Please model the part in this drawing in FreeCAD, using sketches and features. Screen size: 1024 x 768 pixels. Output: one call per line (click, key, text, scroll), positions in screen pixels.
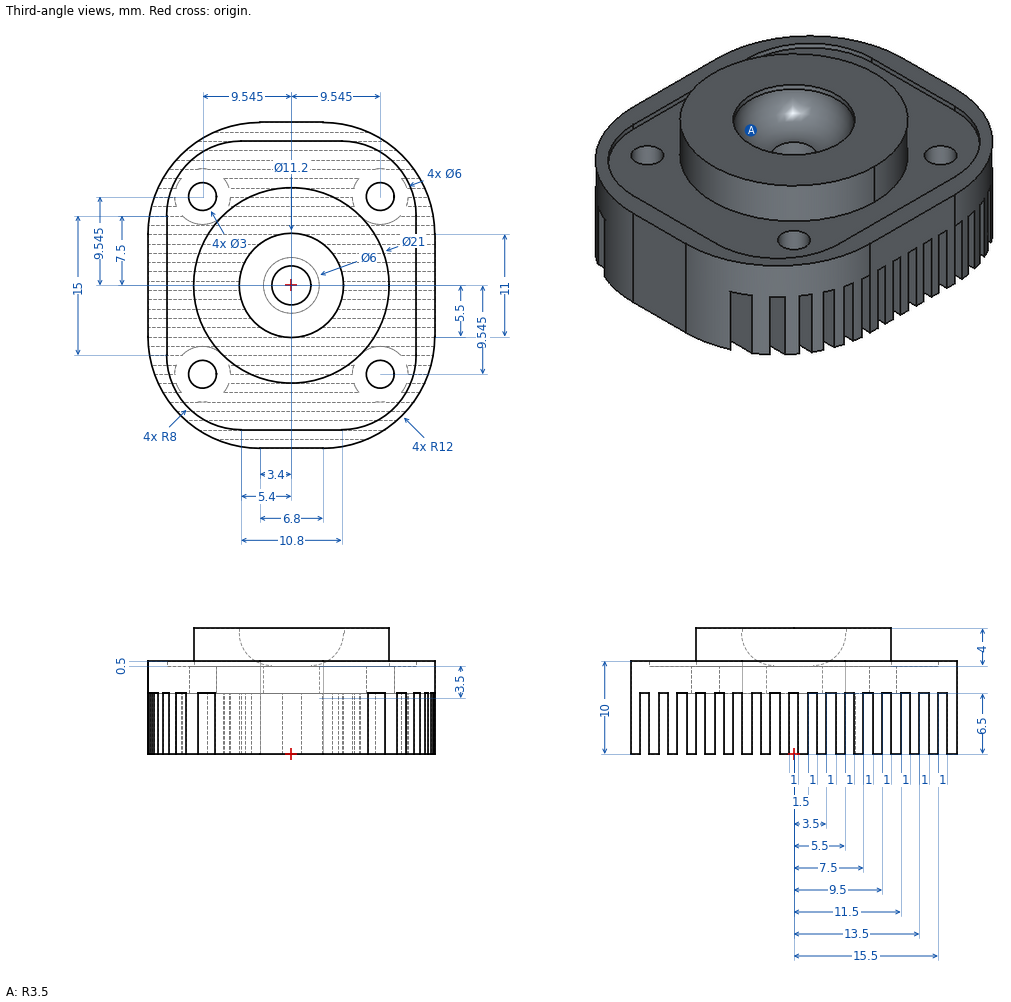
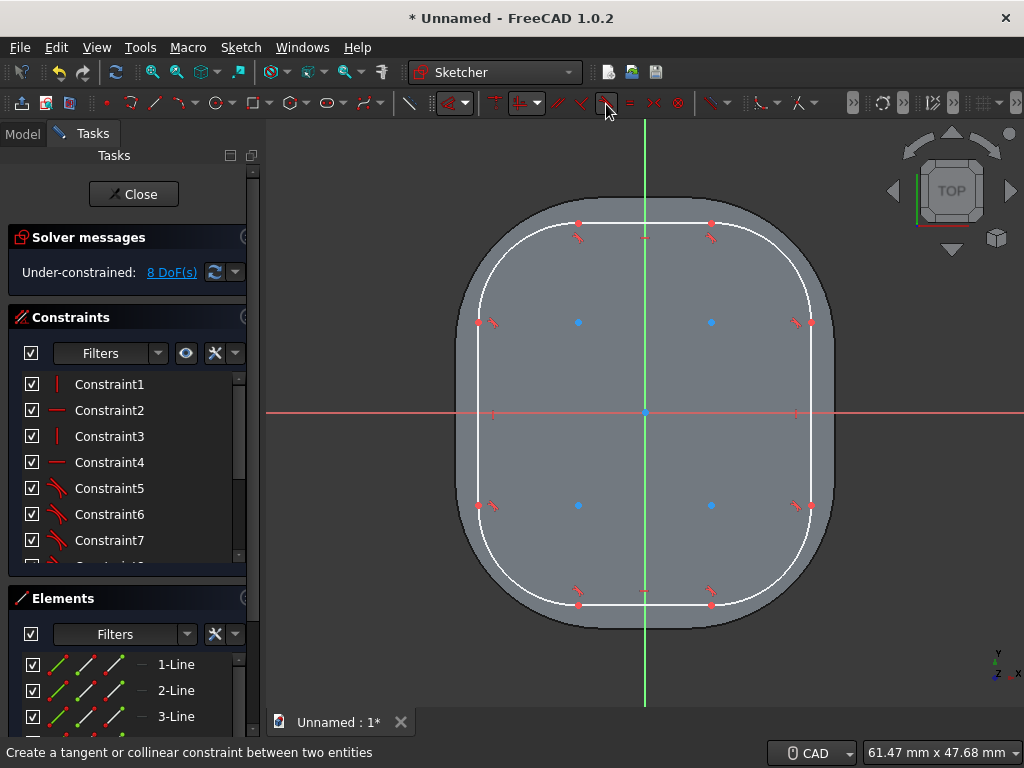
click(489, 551)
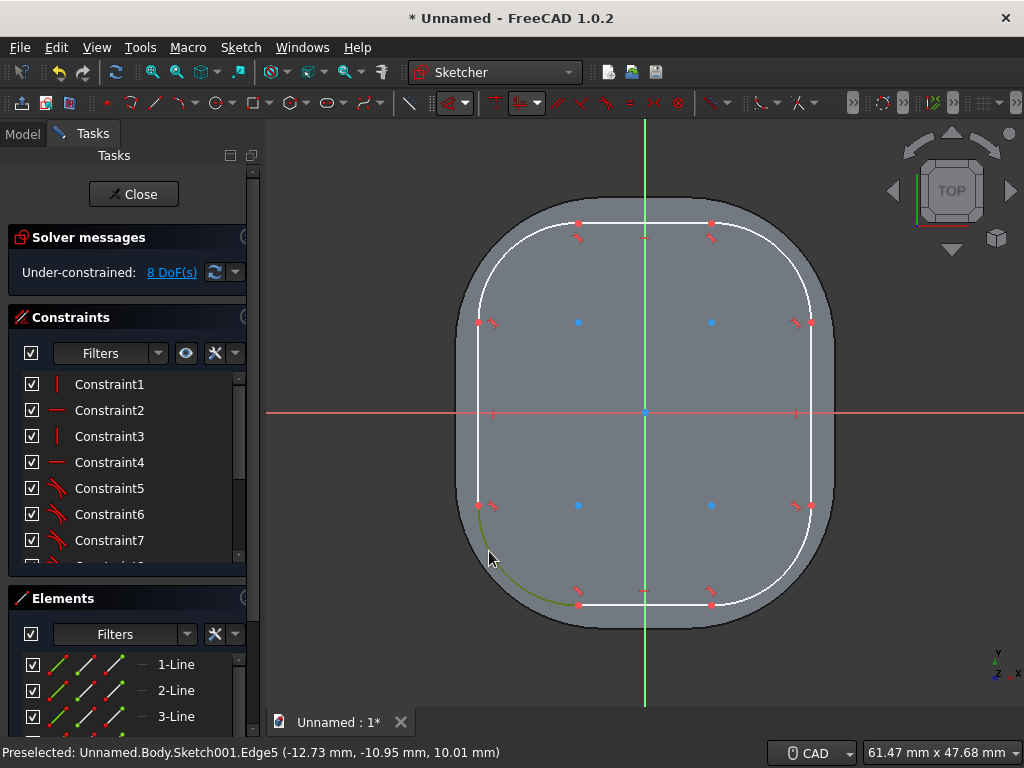
click(757, 595)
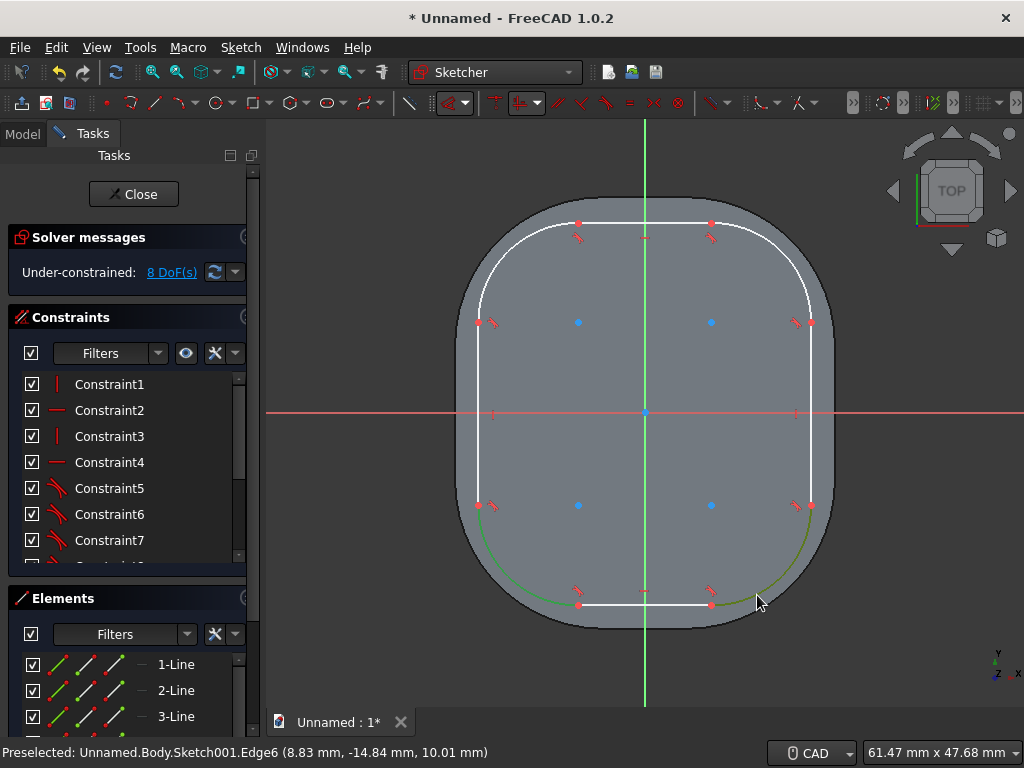
click(800, 277)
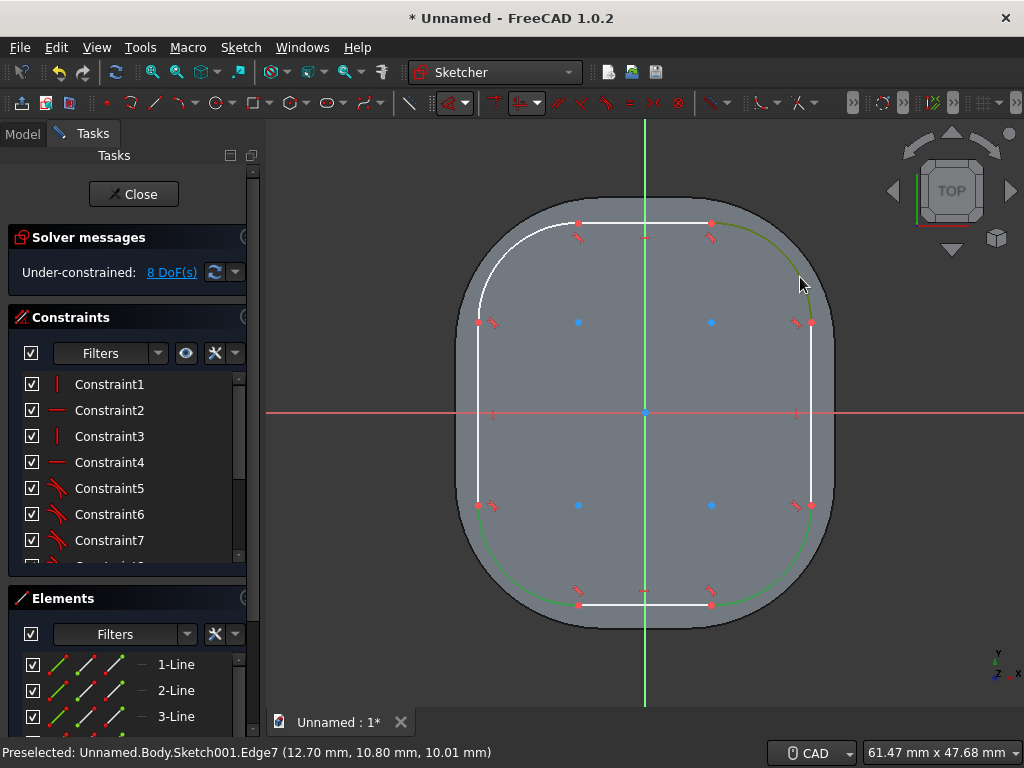
click(533, 234)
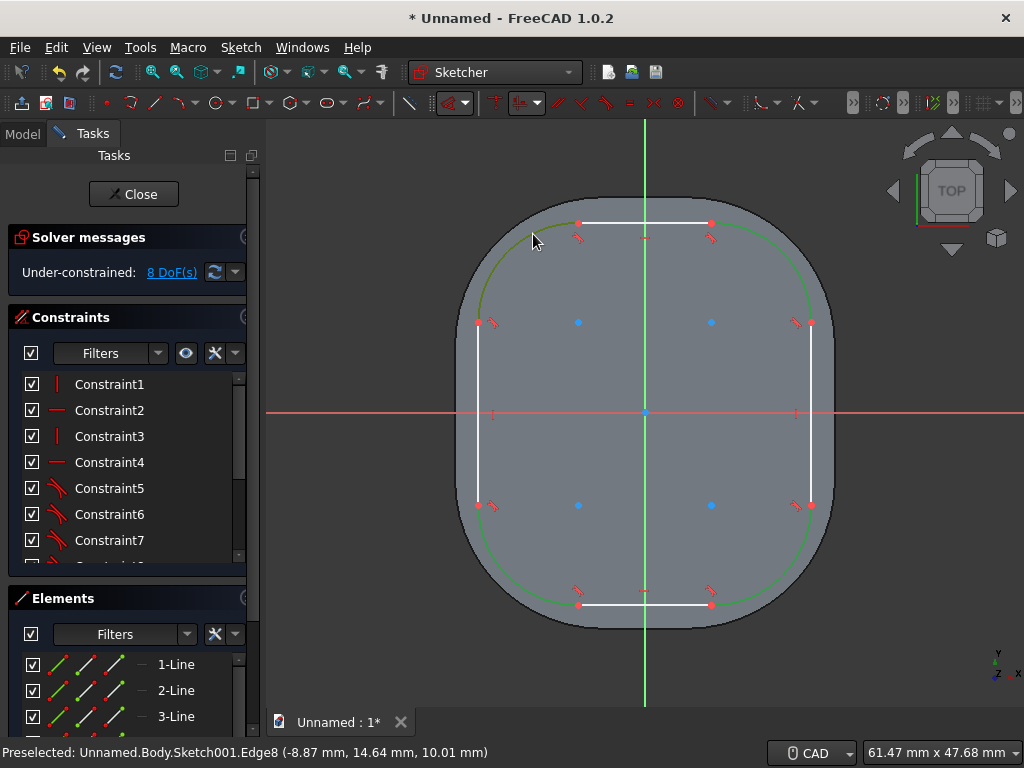
click(630, 104)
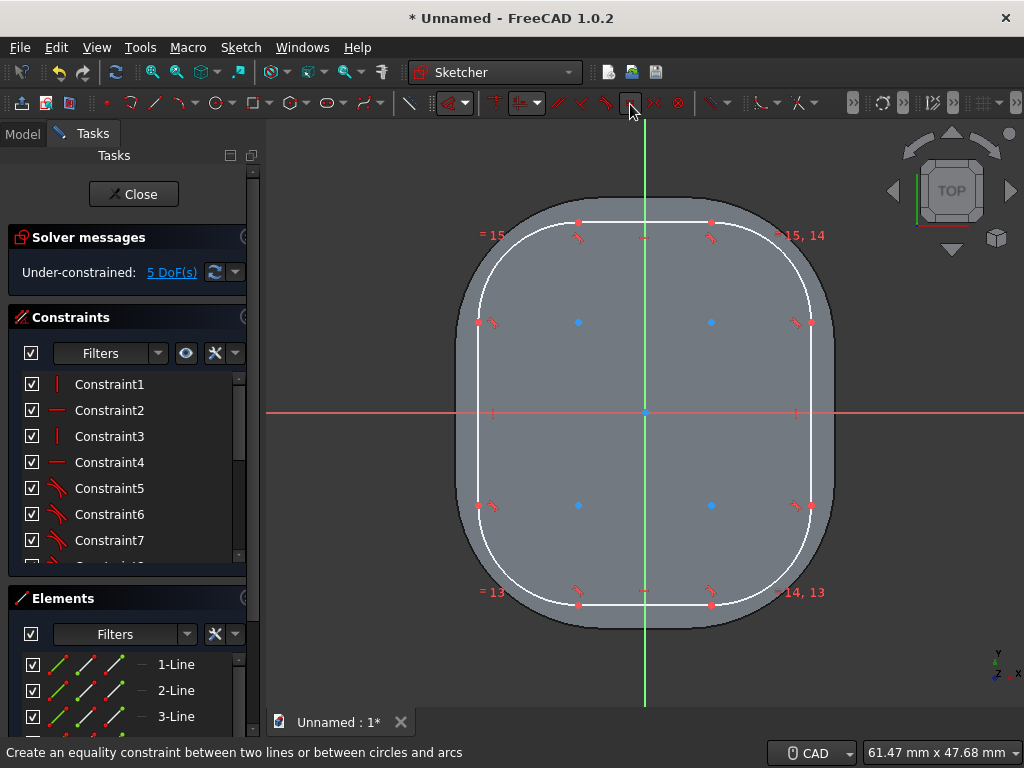
click(489, 551)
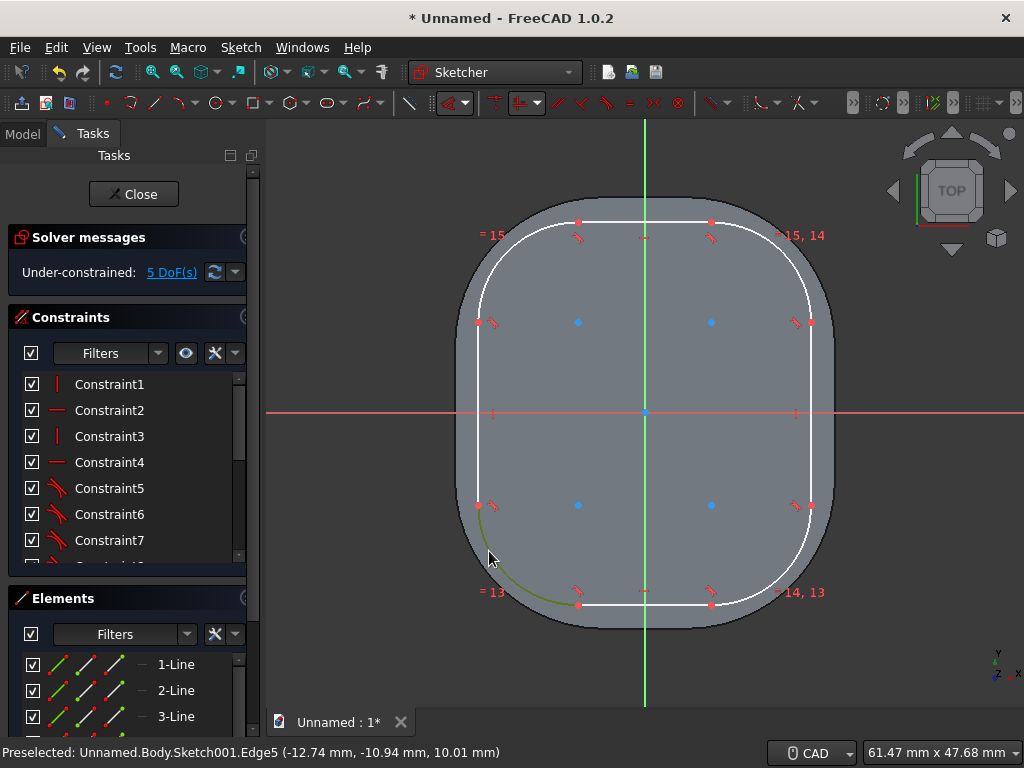
click(468, 104)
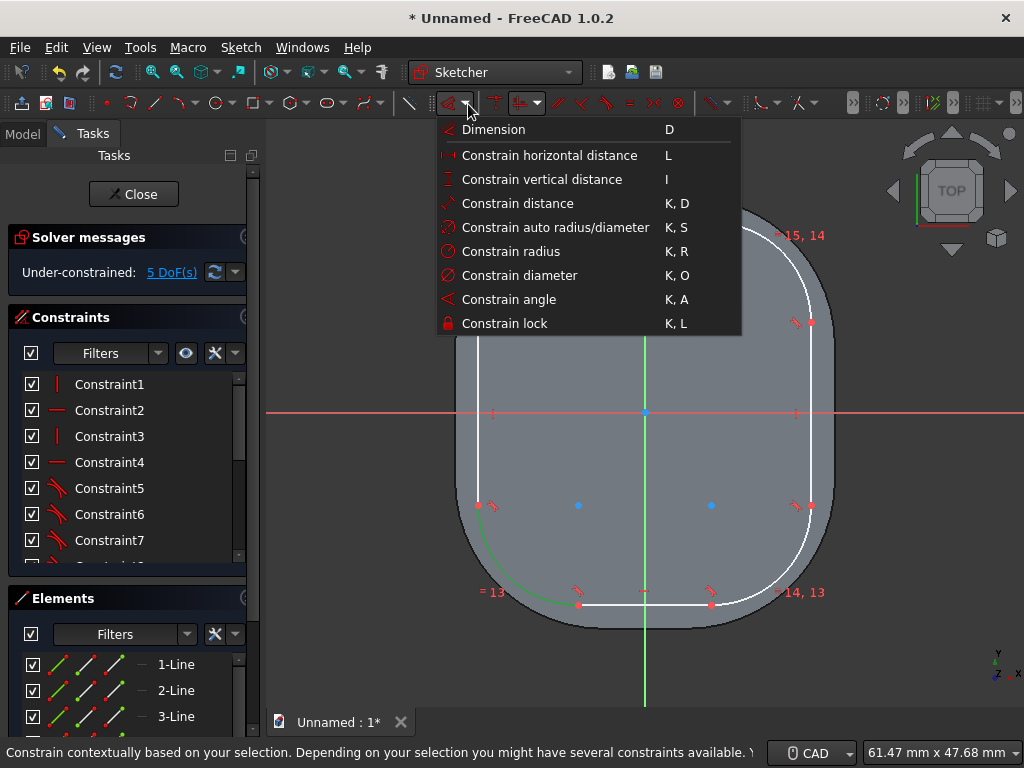
click(589, 251)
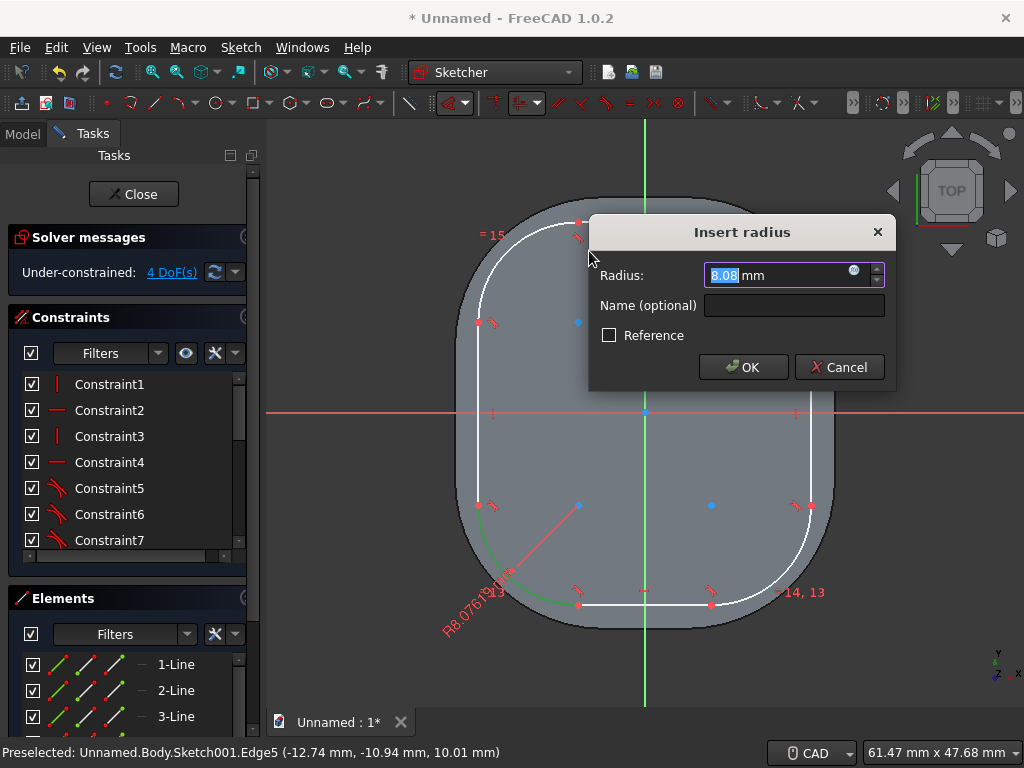
text(8)
key(Return)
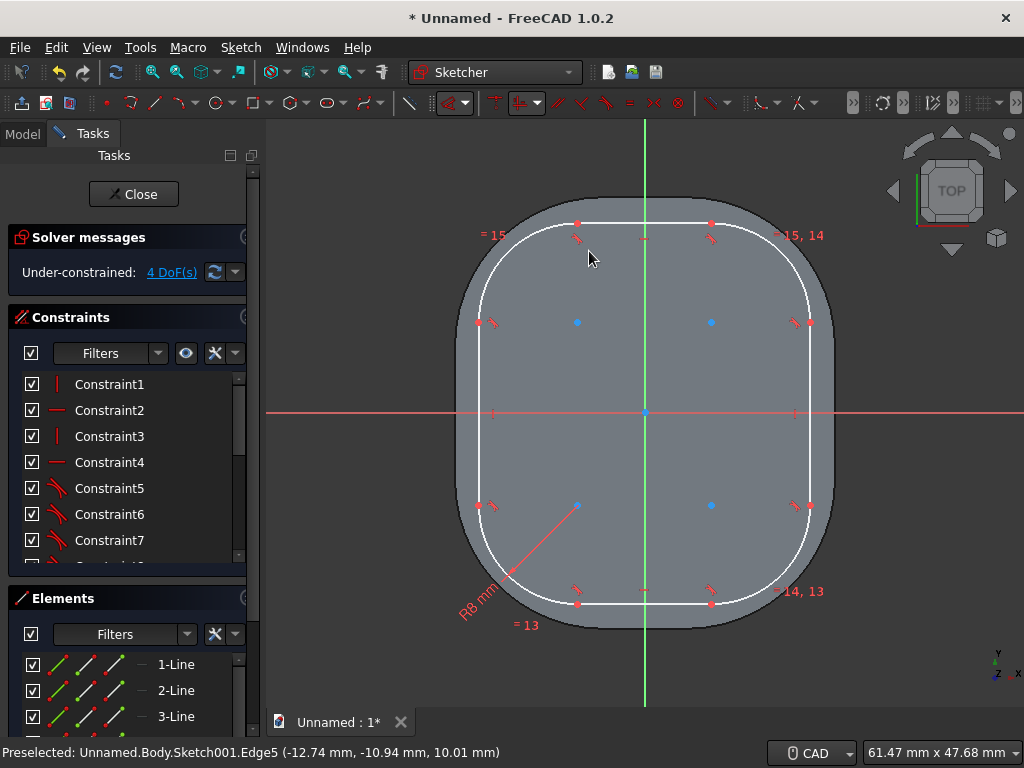
click(479, 377)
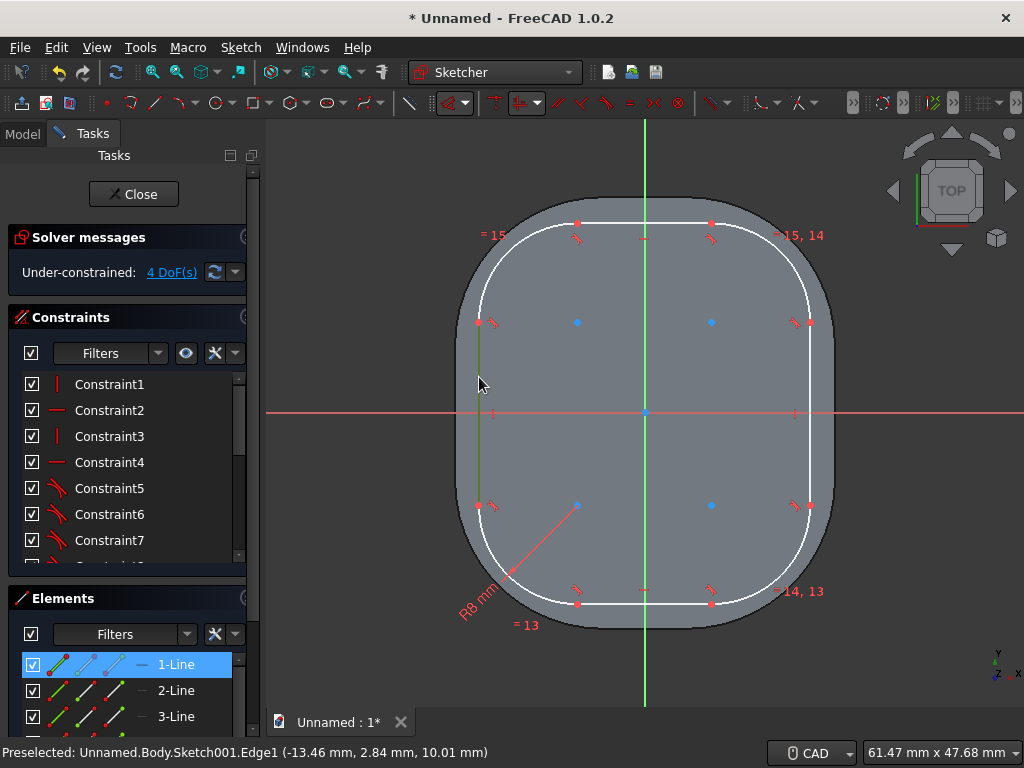
click(468, 104)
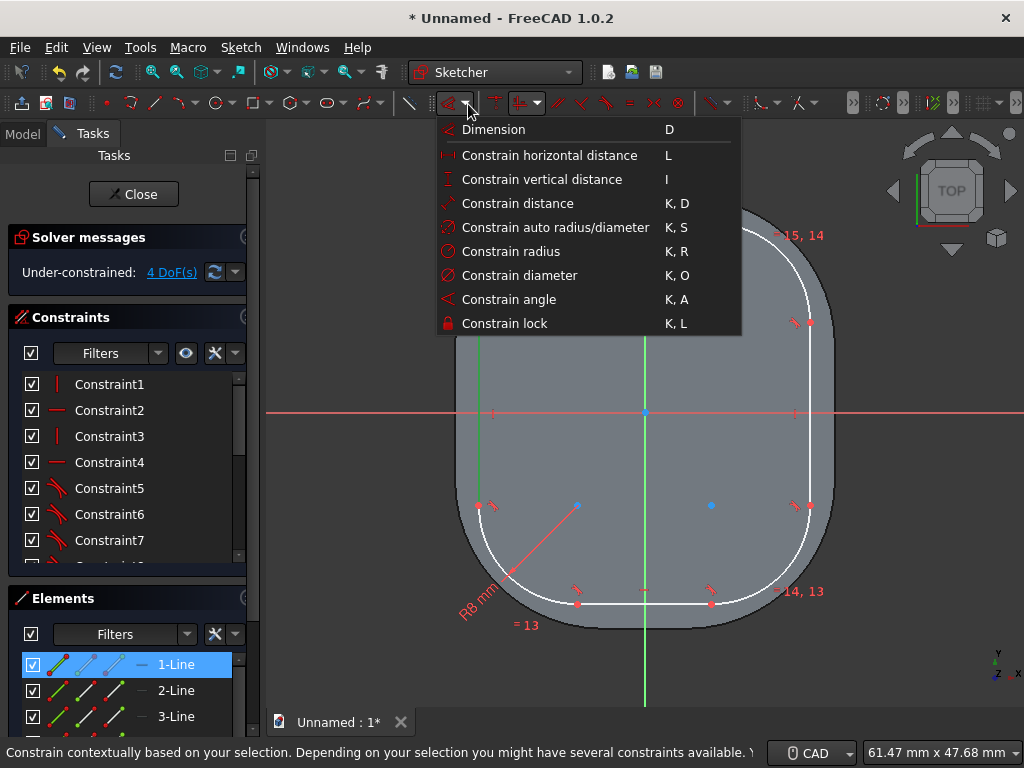
click(589, 179)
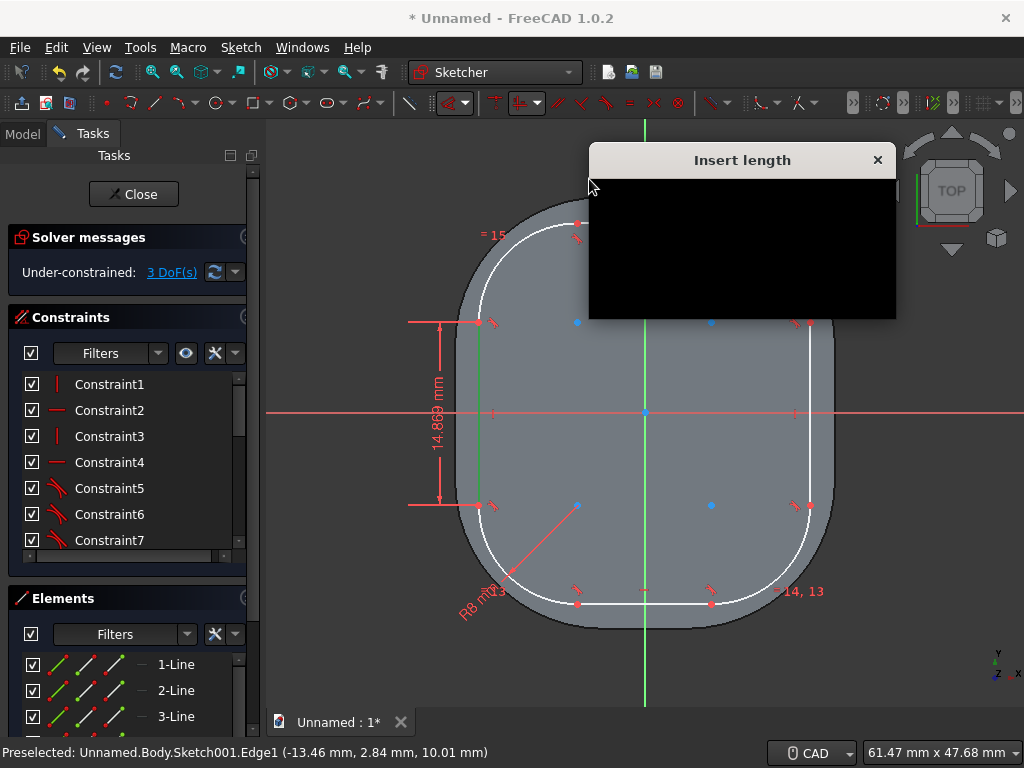
text(15)
key(Return)